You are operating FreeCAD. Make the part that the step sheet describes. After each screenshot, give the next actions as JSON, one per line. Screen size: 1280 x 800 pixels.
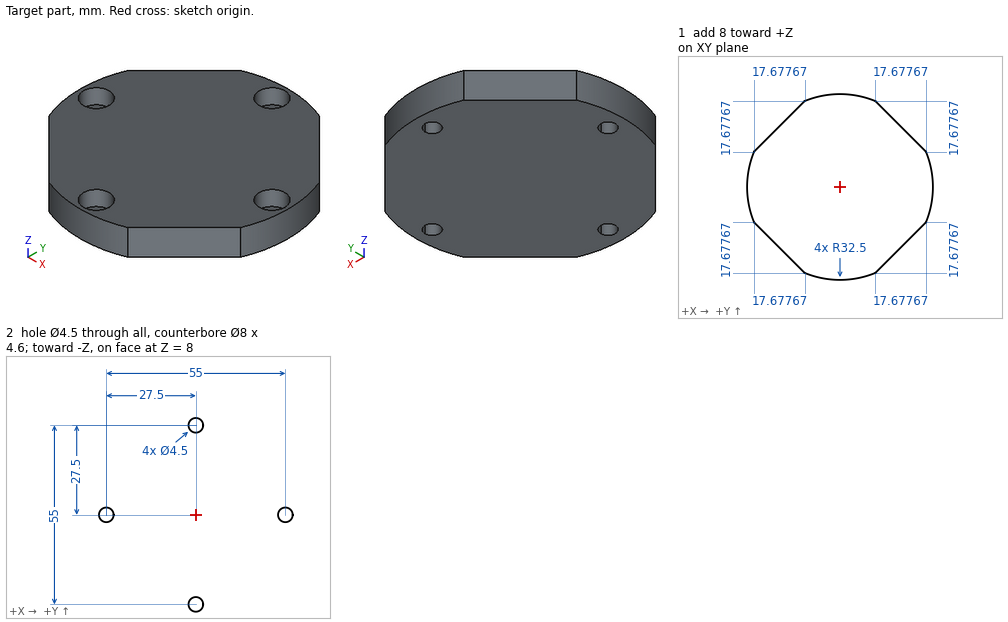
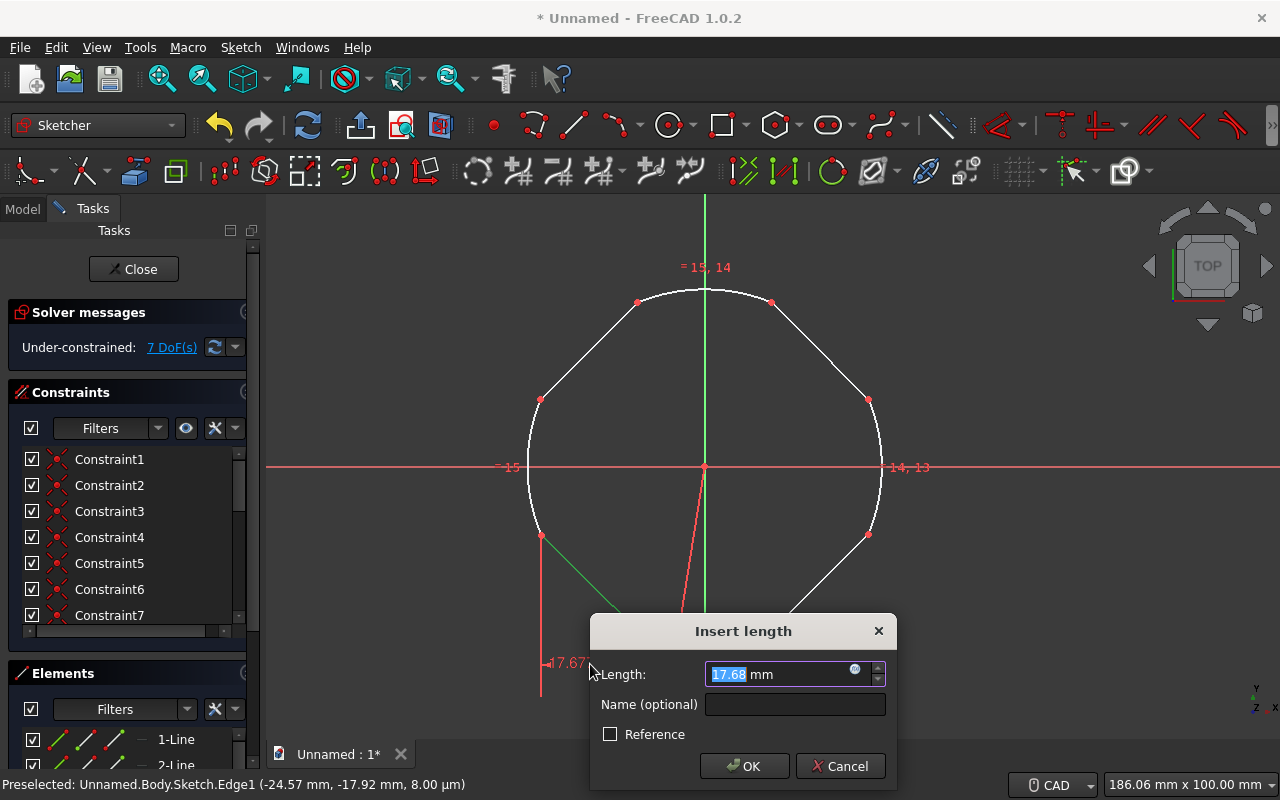
{"action": "type", "text": "17.67767"}
{"action": "key", "text": "Return"}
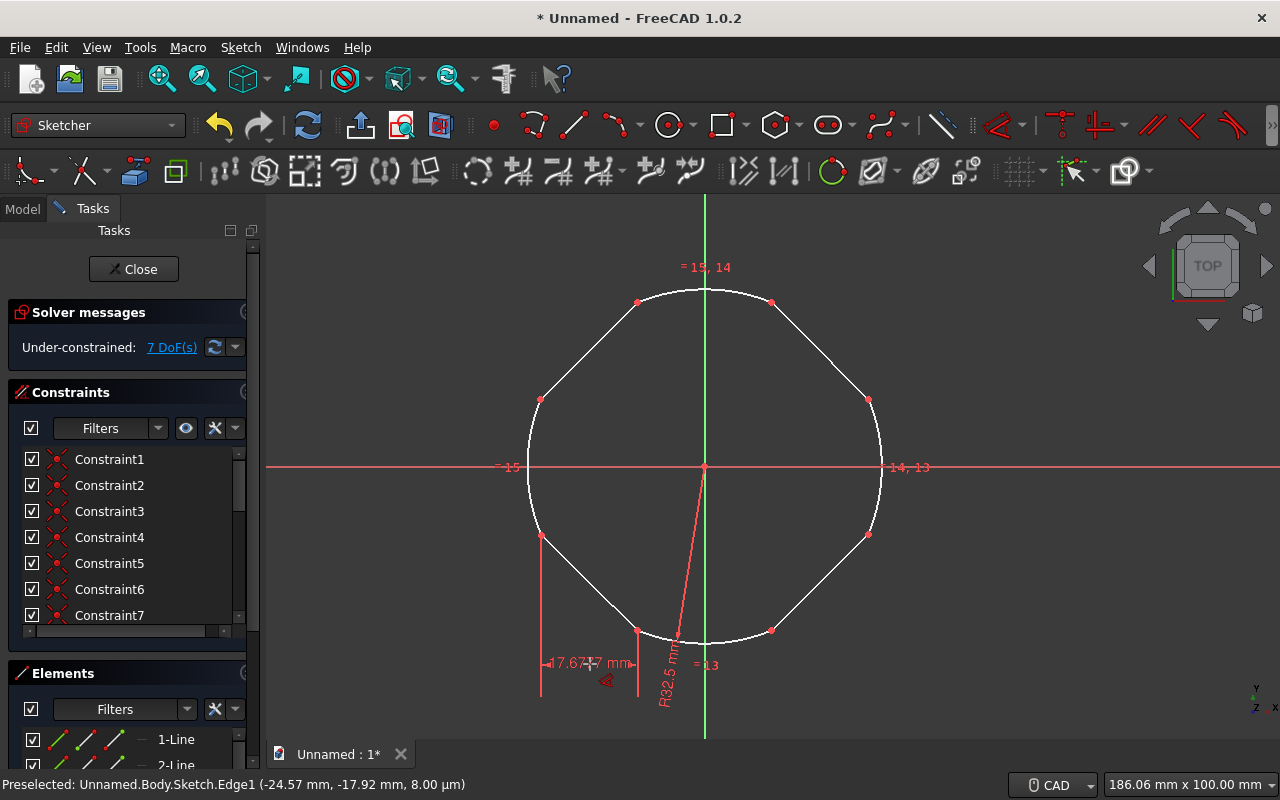
{"action": "left_click", "coordinate": [570, 564]}
{"action": "left_click", "coordinate": [507, 583]}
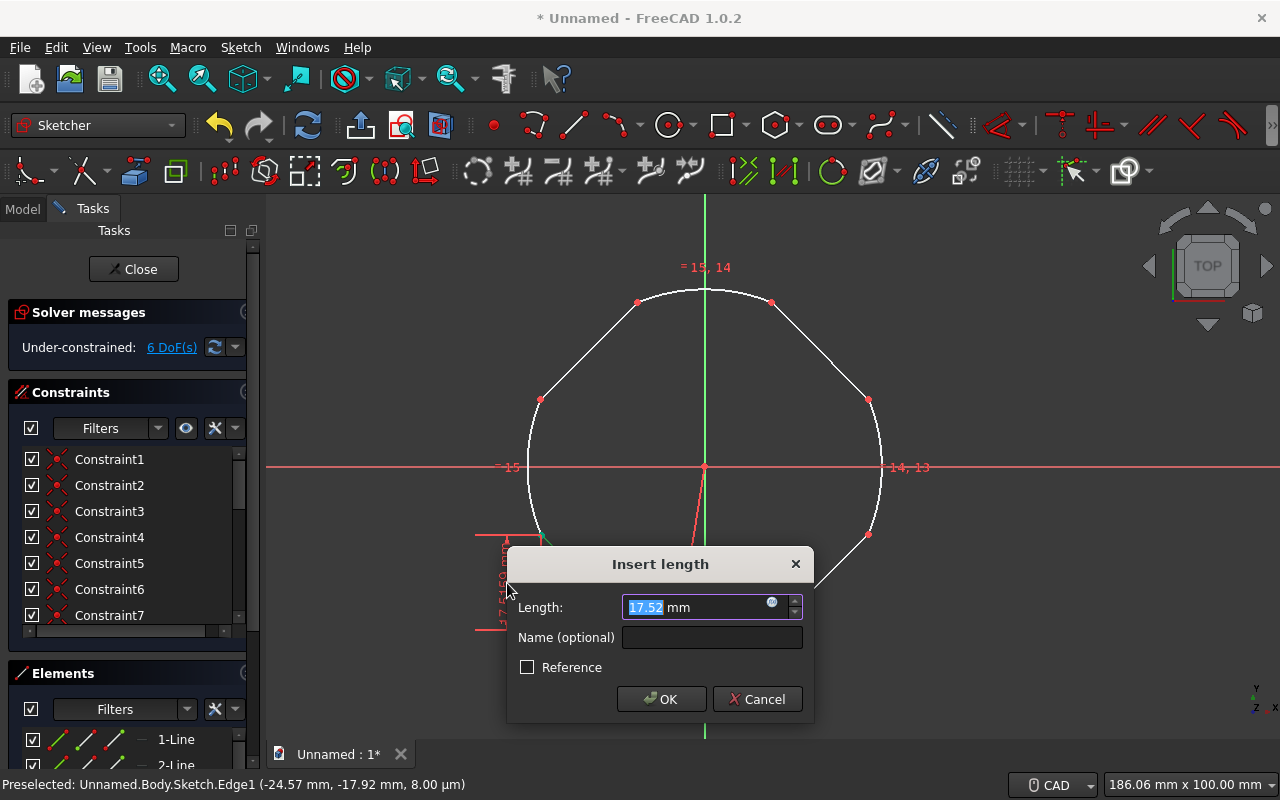
{"action": "type", "text": "17.67767"}
{"action": "key", "text": "Return"}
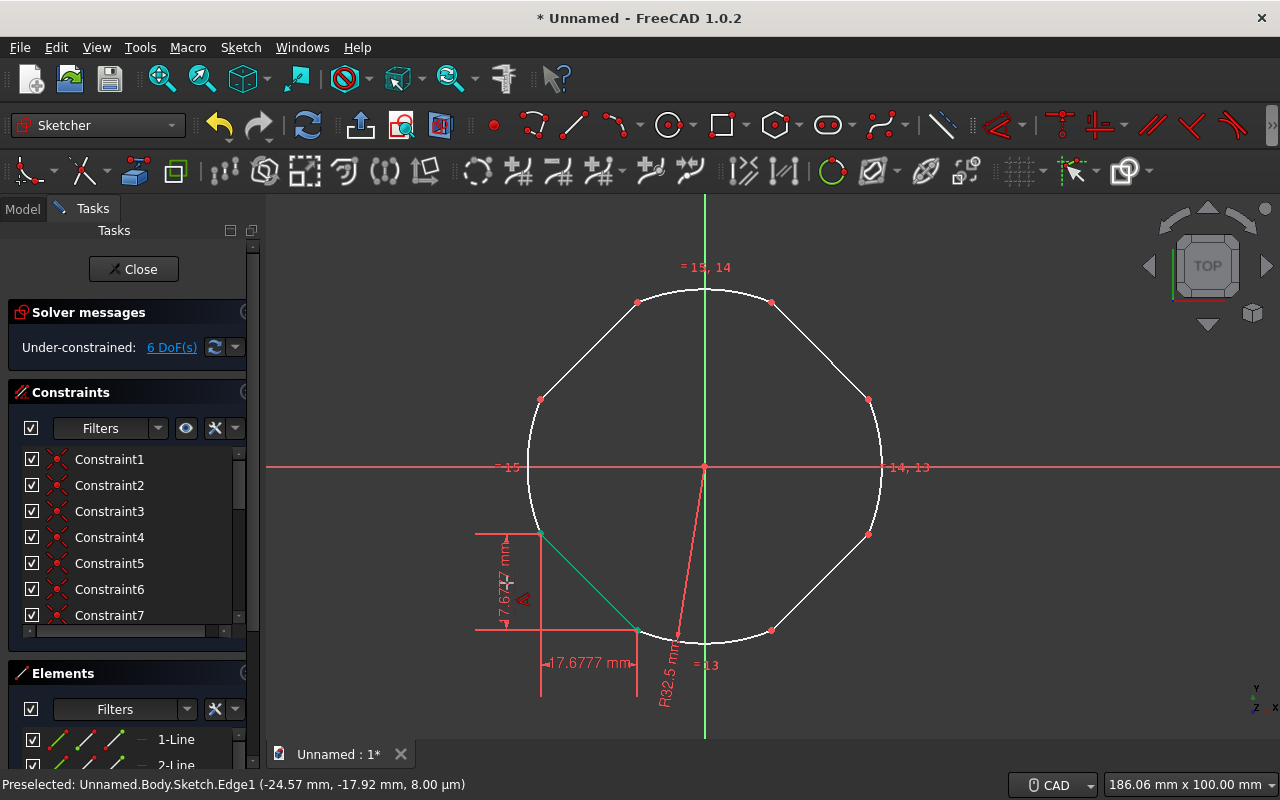
{"action": "left_click", "coordinate": [801, 602]}
{"action": "left_click", "coordinate": [820, 664]}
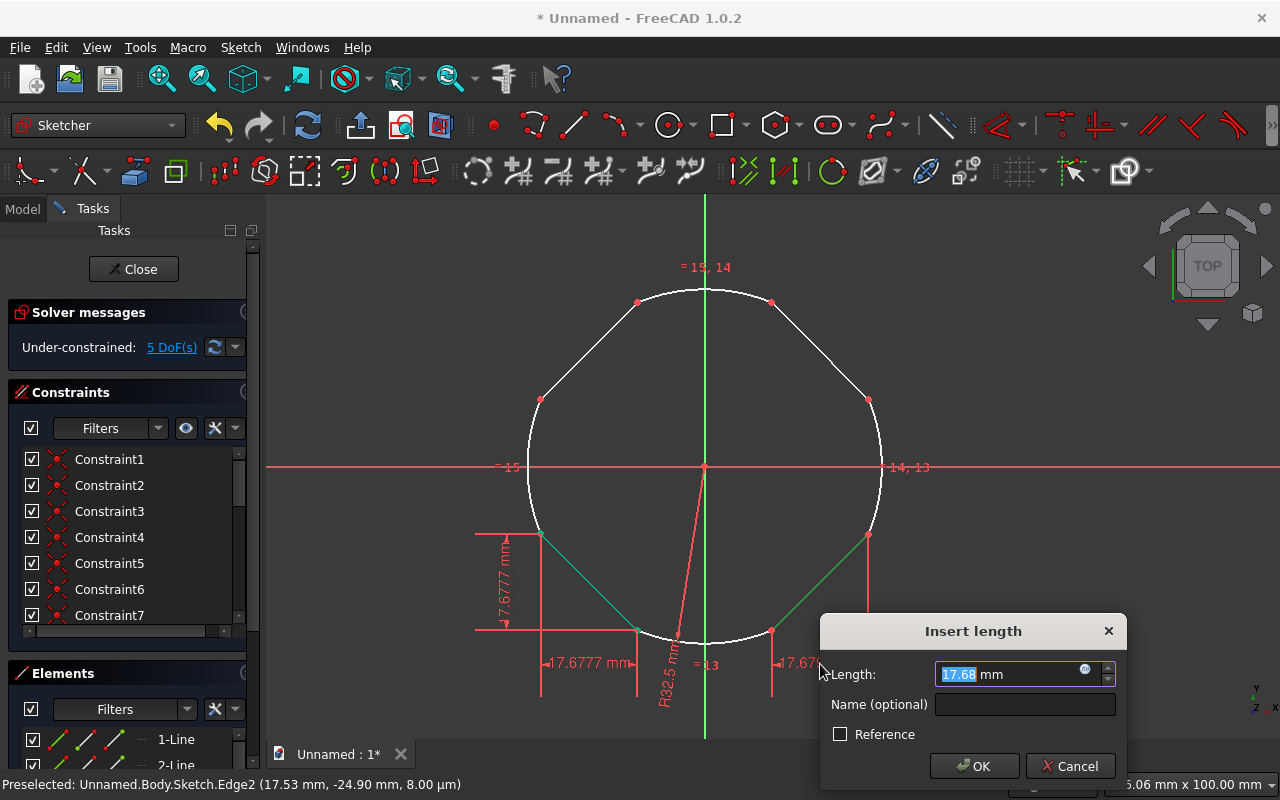
{"action": "type", "text": "17.67767"}
{"action": "key", "text": "Return"}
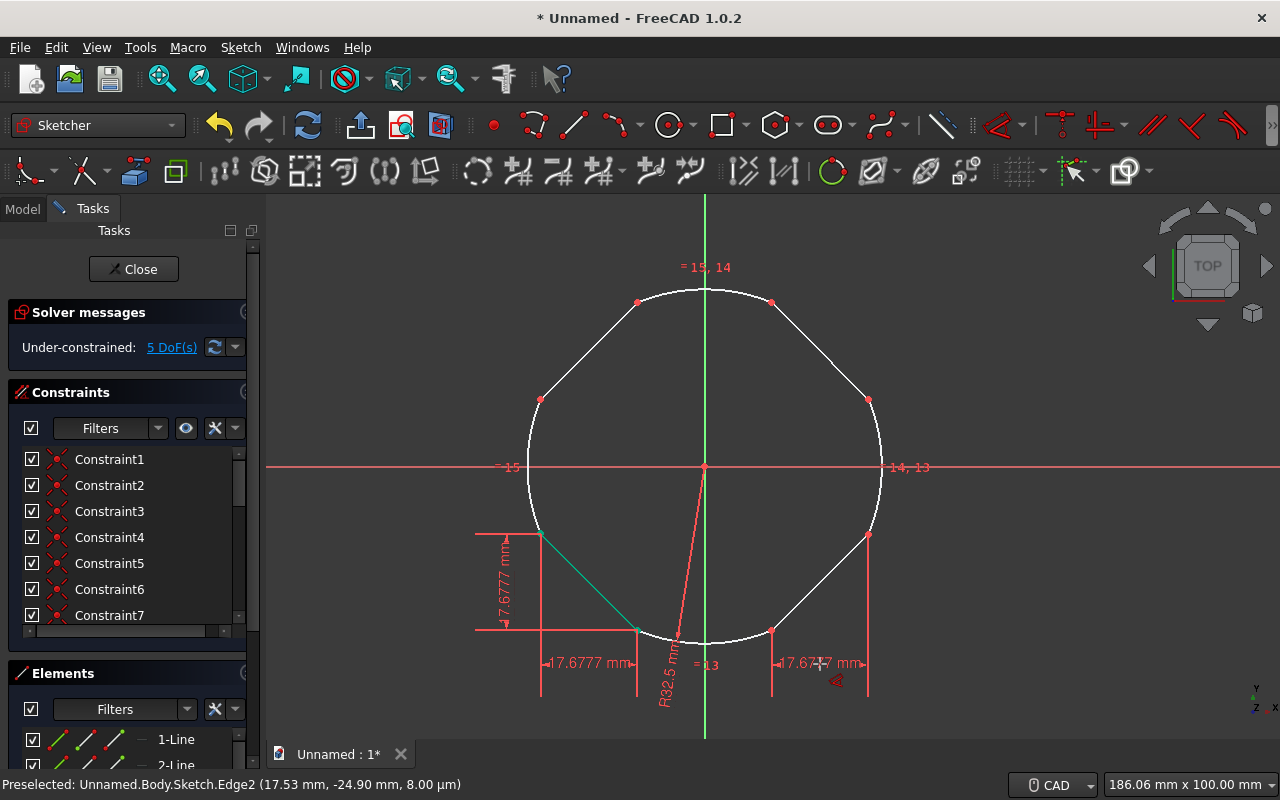
{"action": "left_click", "coordinate": [801, 602]}
{"action": "left_click", "coordinate": [902, 583]}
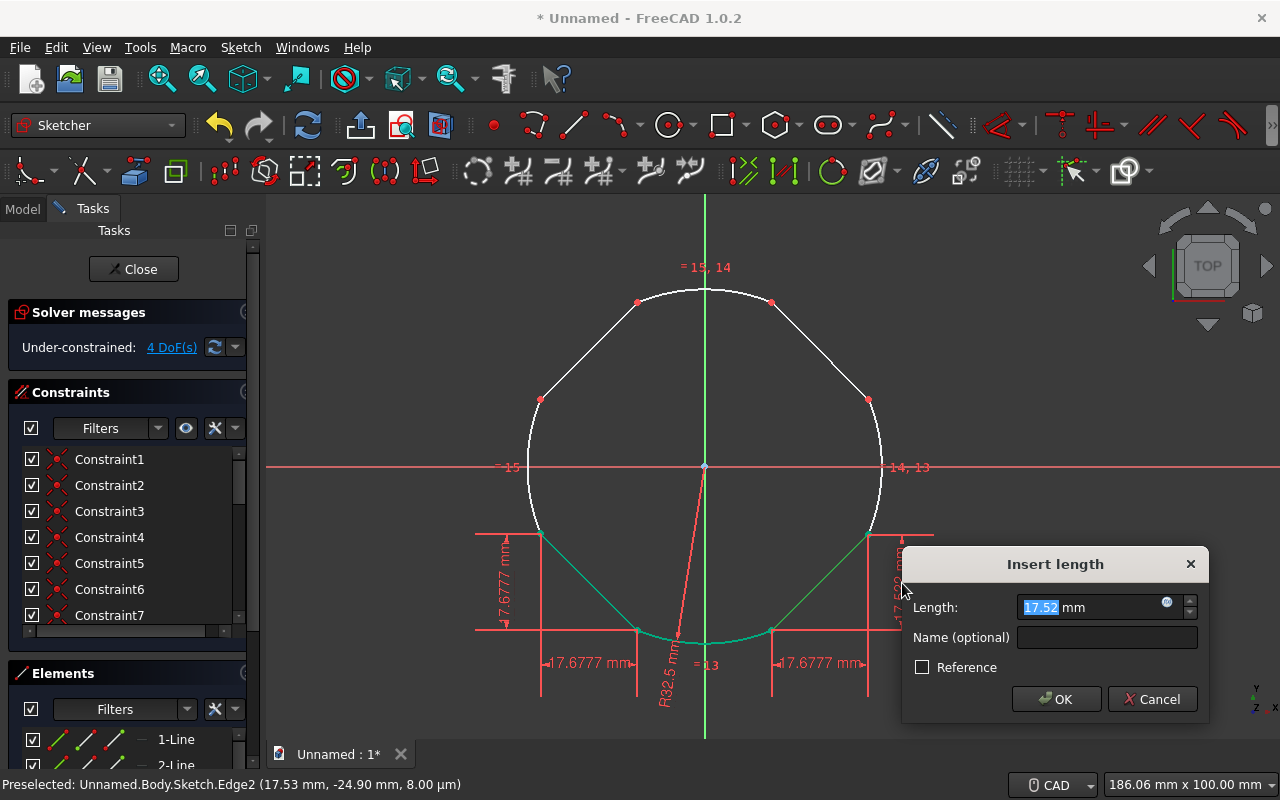
{"action": "type", "text": "17.67767"}
{"action": "key", "text": "Return"}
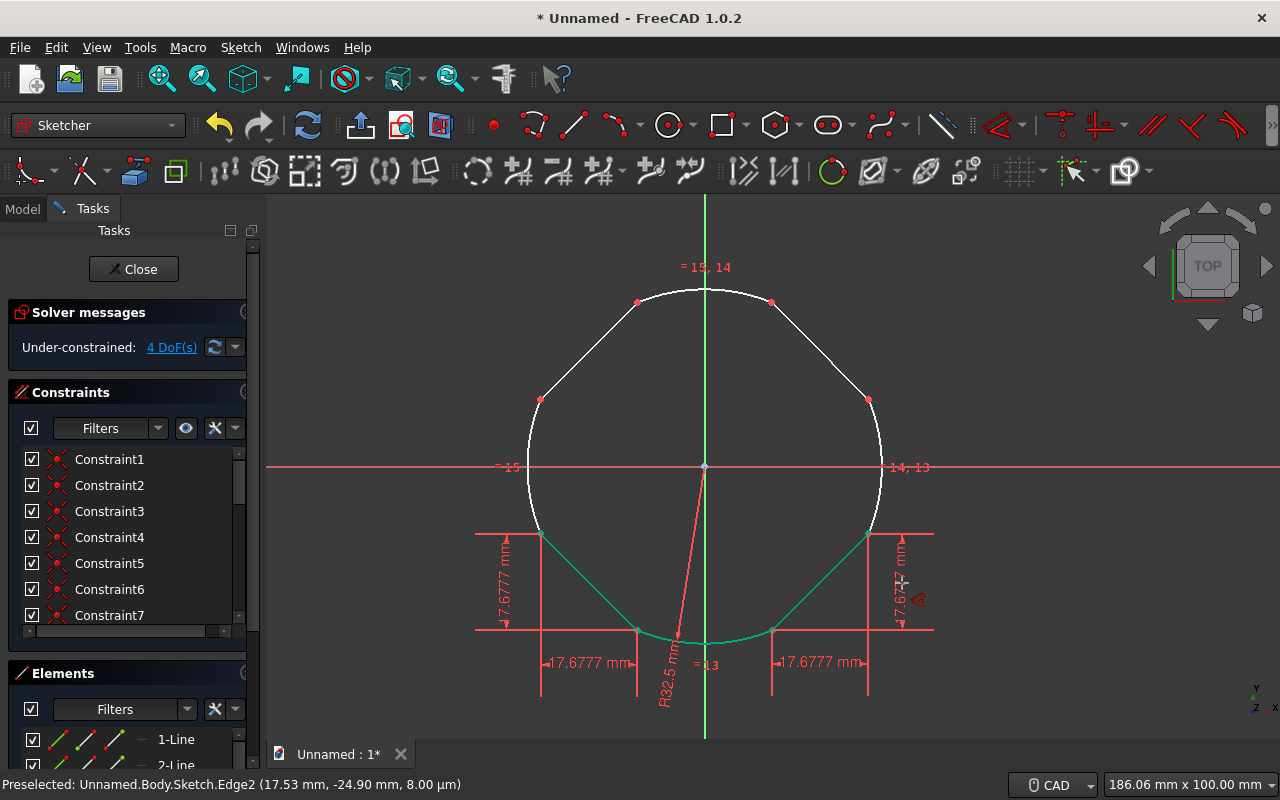
{"action": "left_click", "coordinate": [840, 371]}
{"action": "left_click", "coordinate": [820, 269]}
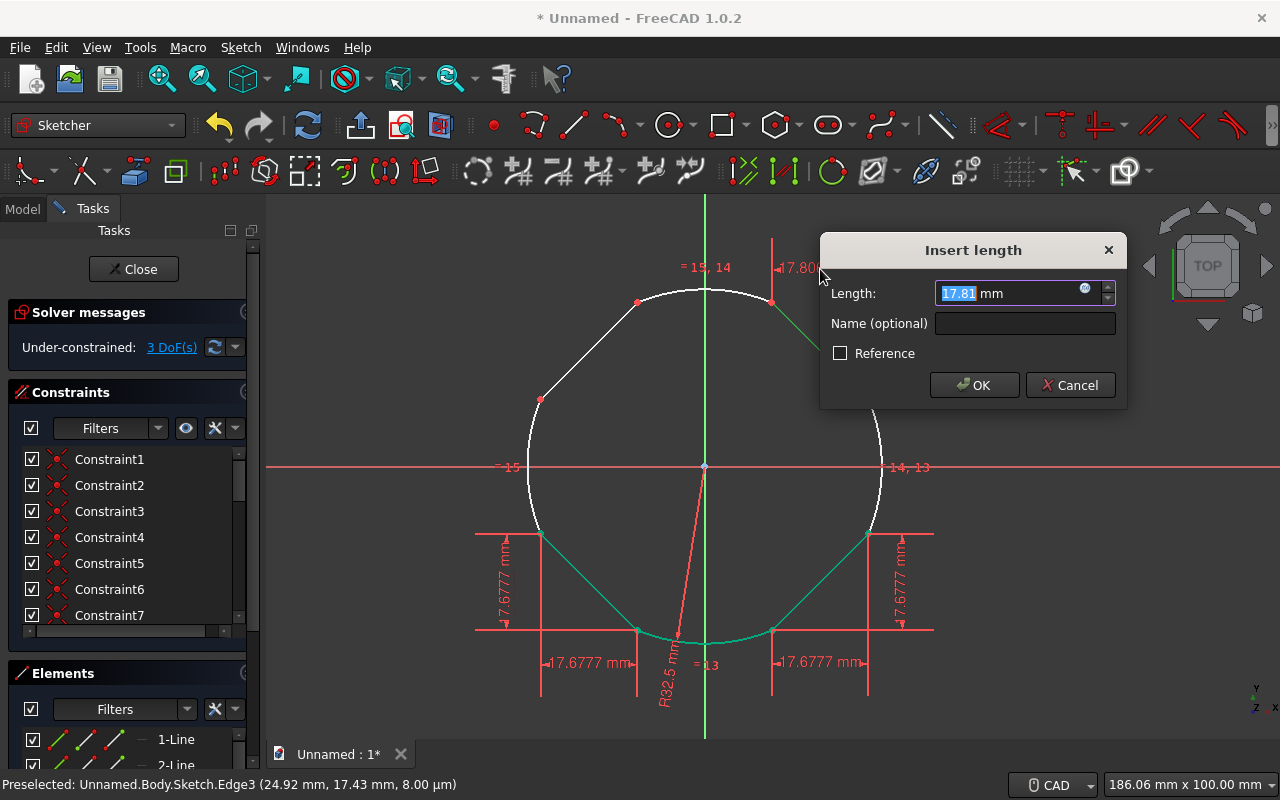
{"action": "type", "text": "17.67767"}
{"action": "key", "text": "Return"}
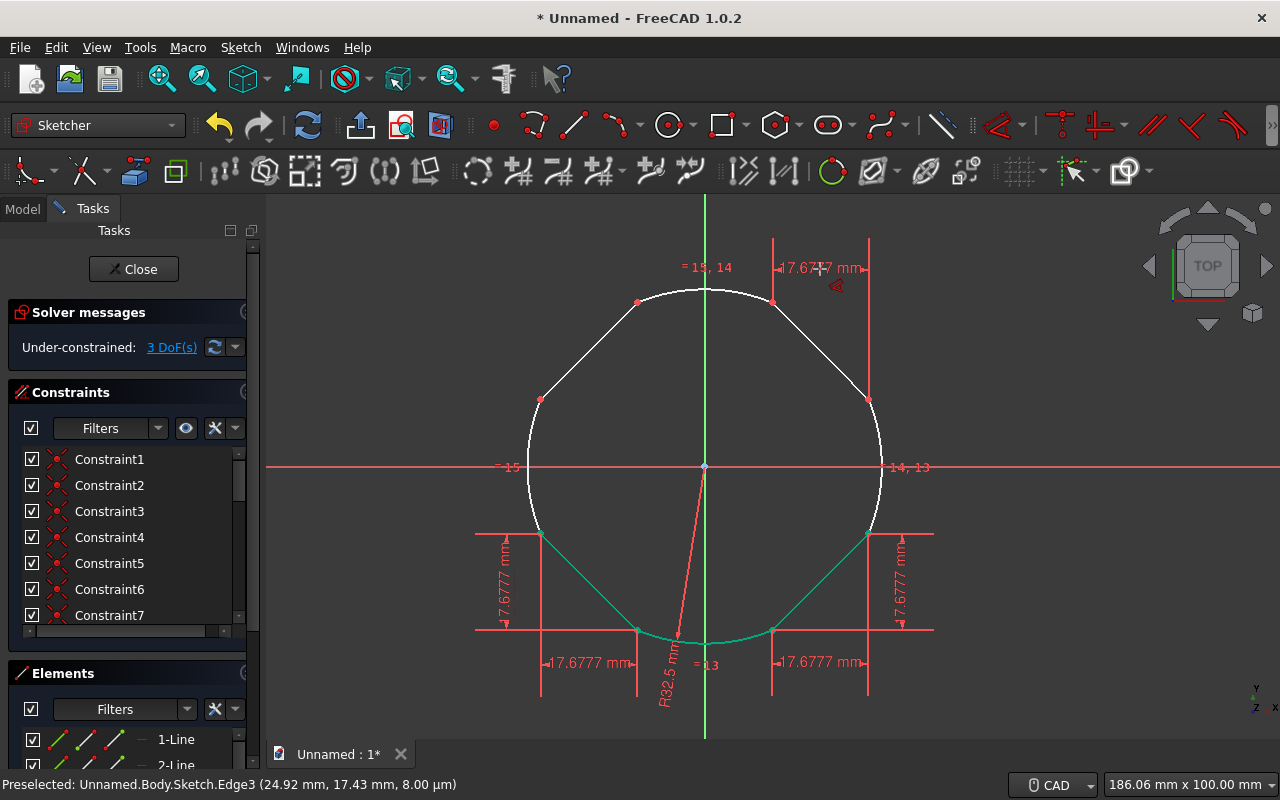
{"action": "left_click", "coordinate": [840, 371]}
{"action": "left_click", "coordinate": [903, 351]}